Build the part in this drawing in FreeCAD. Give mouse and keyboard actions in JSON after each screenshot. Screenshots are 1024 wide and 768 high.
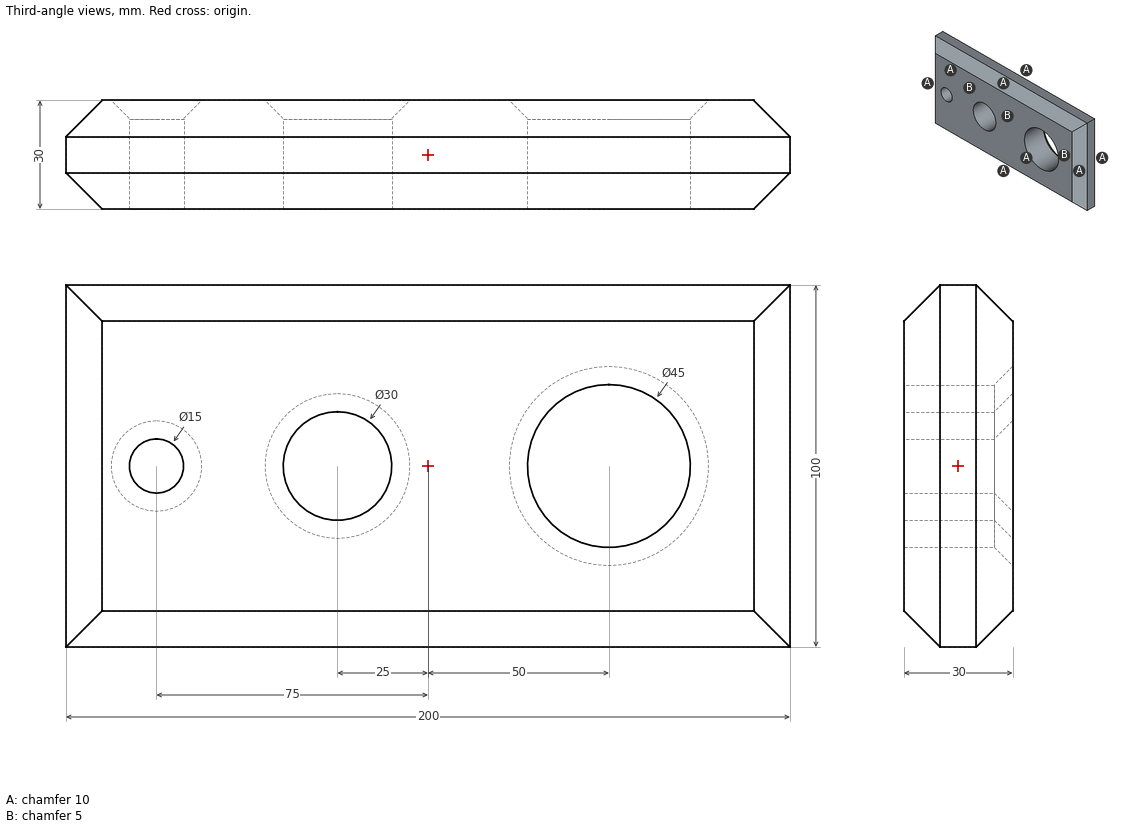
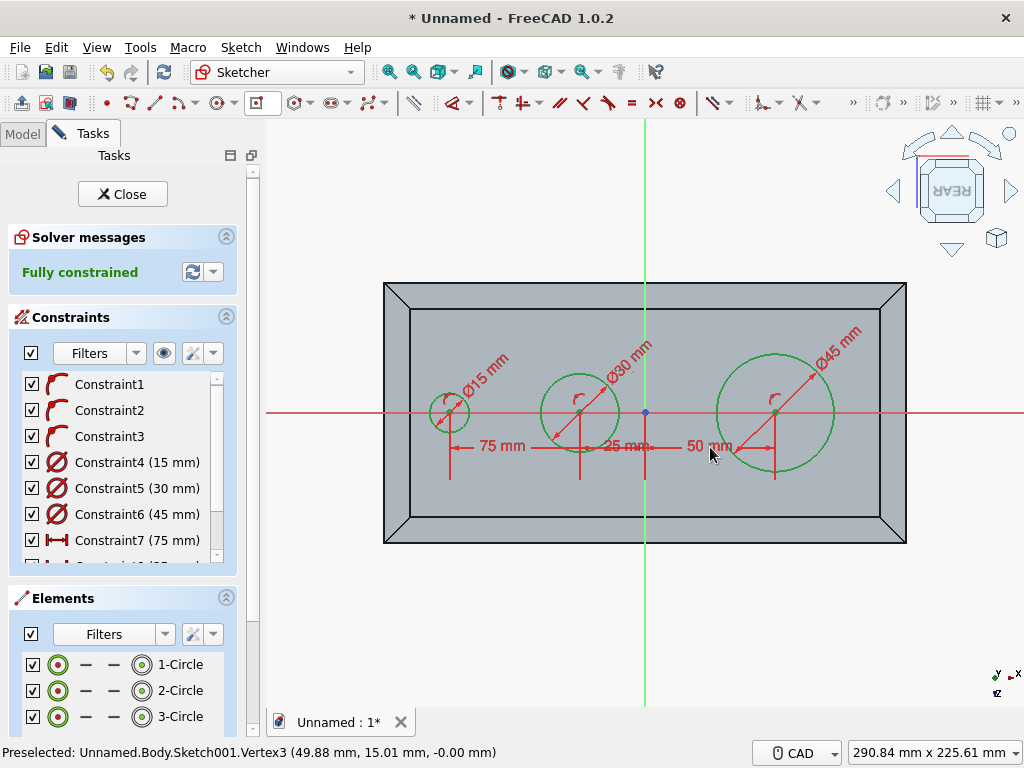
{"action": "left_click", "coordinate": [123, 194]}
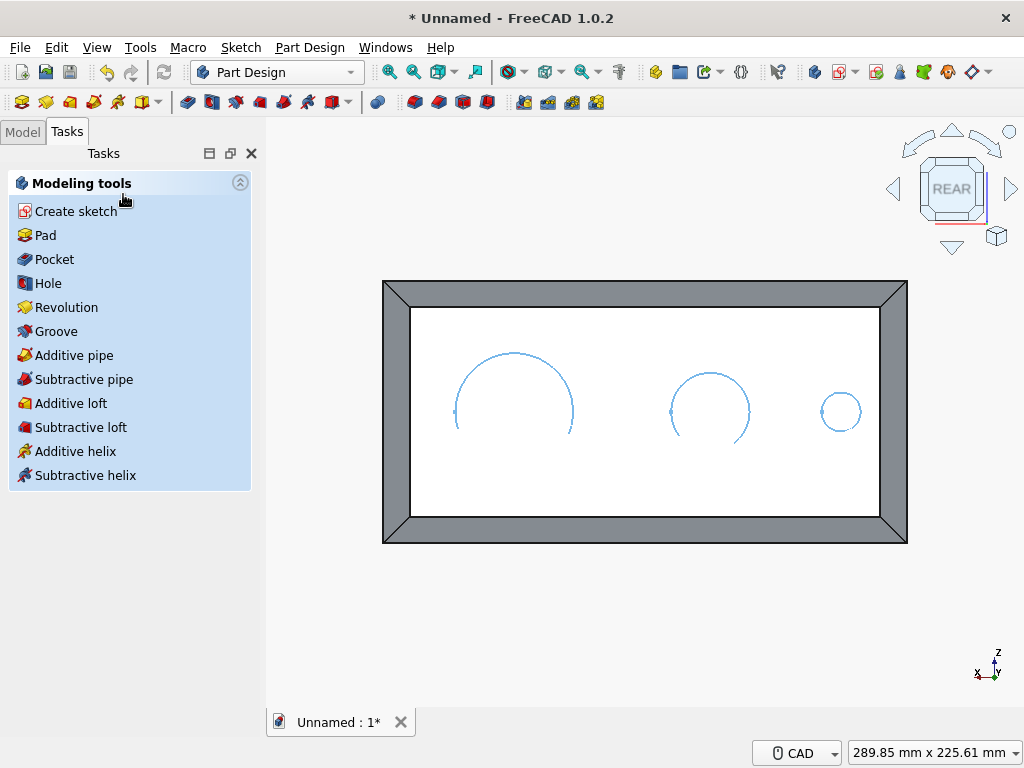
{"action": "left_click", "coordinate": [188, 102]}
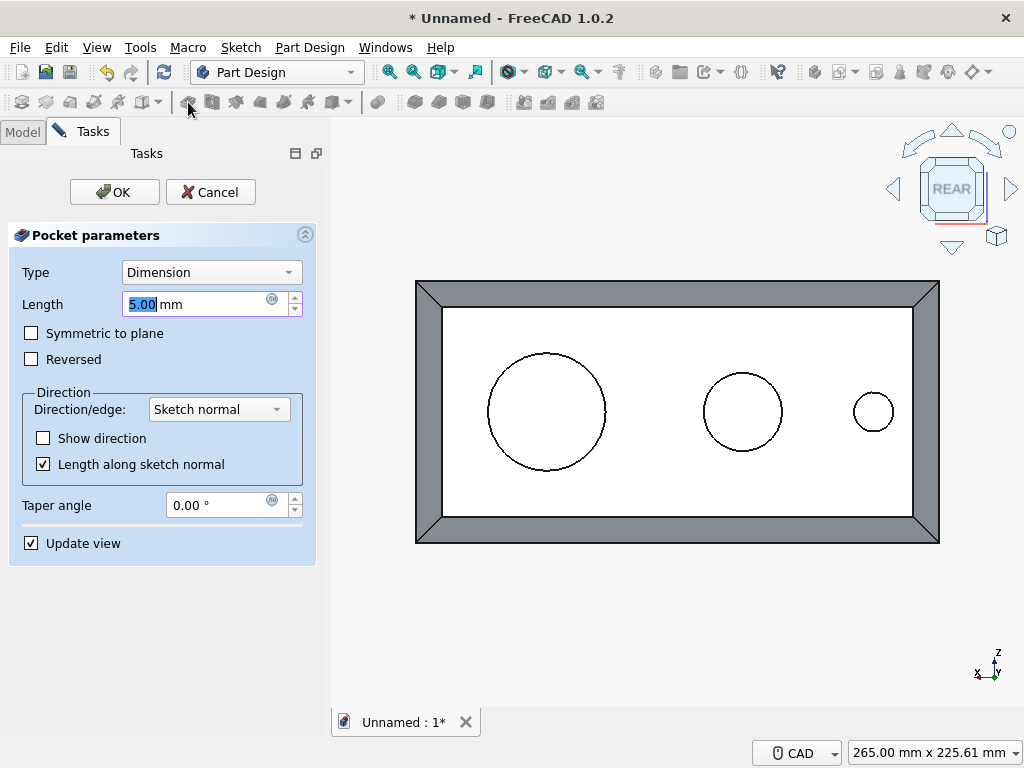
{"action": "type", "text": "30"}
{"action": "key", "text": "Tab"}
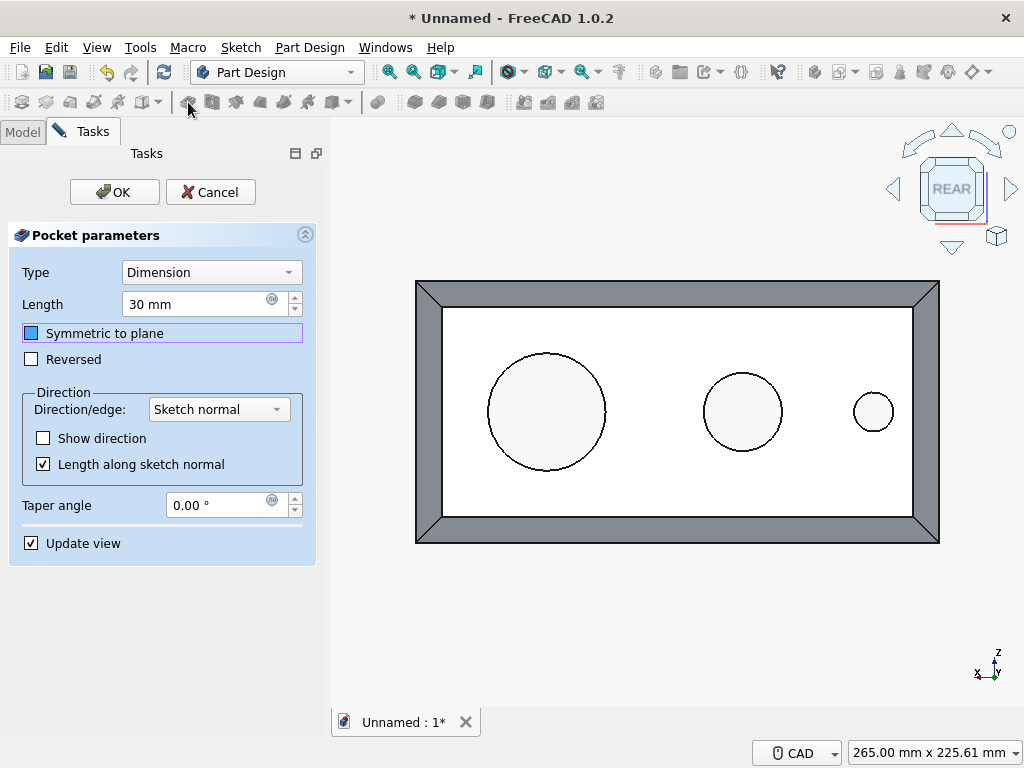
{"action": "left_click", "coordinate": [115, 192]}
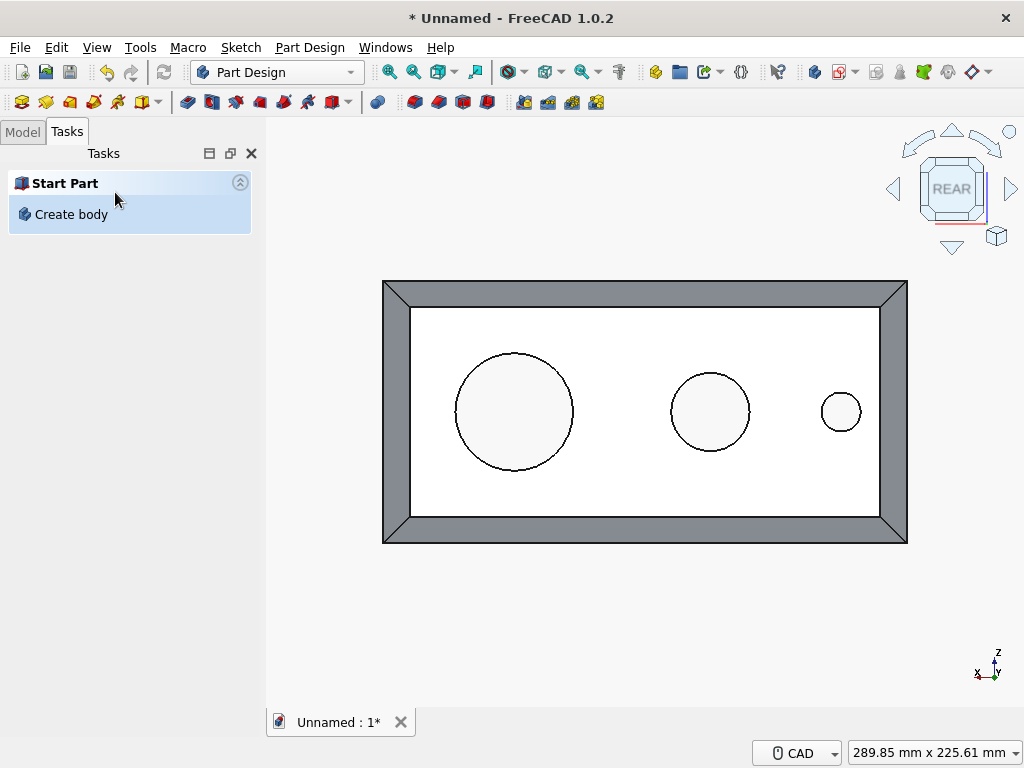
{"action": "left_click", "coordinate": [861, 411]}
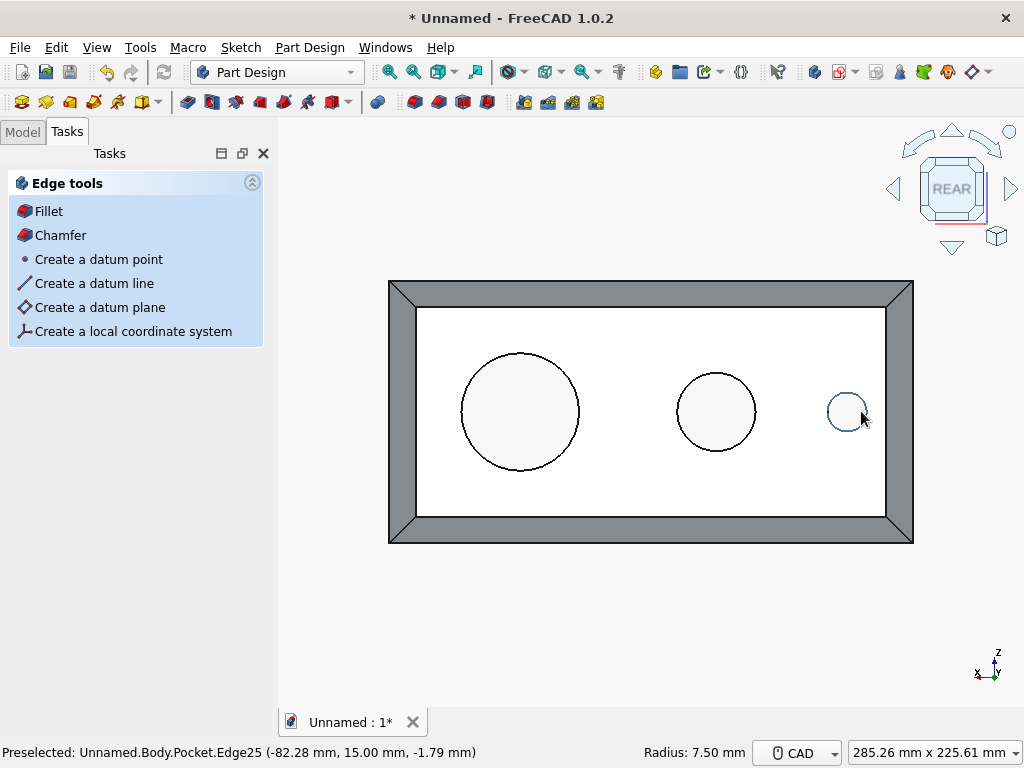
{"action": "left_click", "coordinate": [748, 388], "text": "ctrl"}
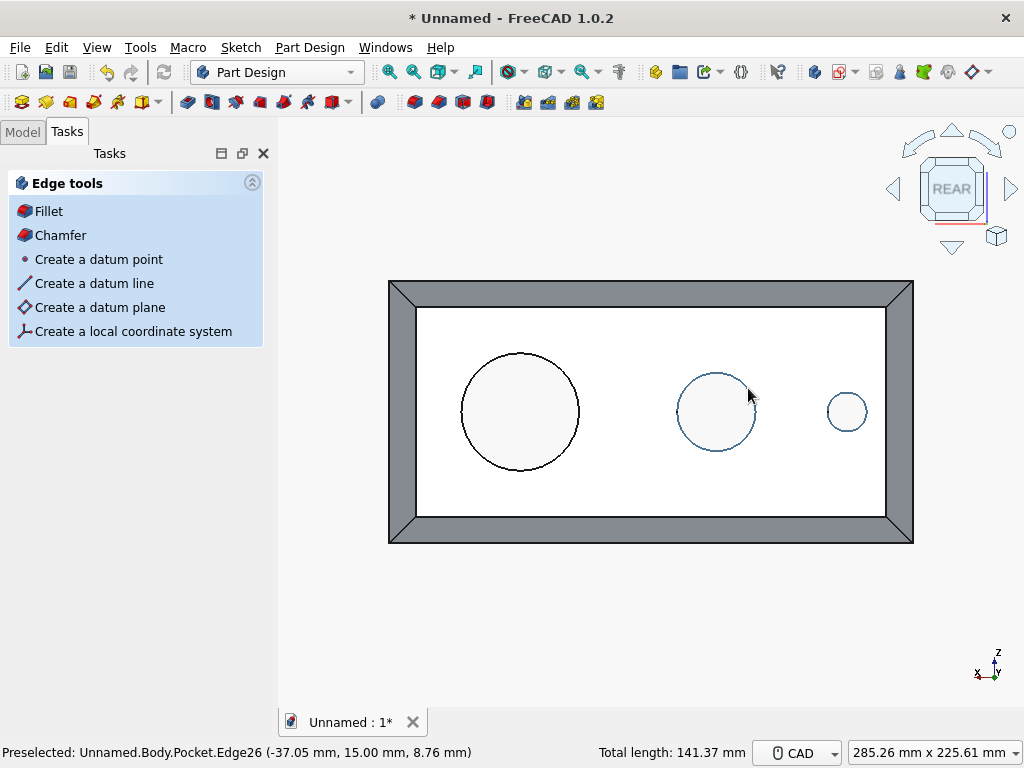
{"action": "left_click", "coordinate": [568, 376], "text": "ctrl"}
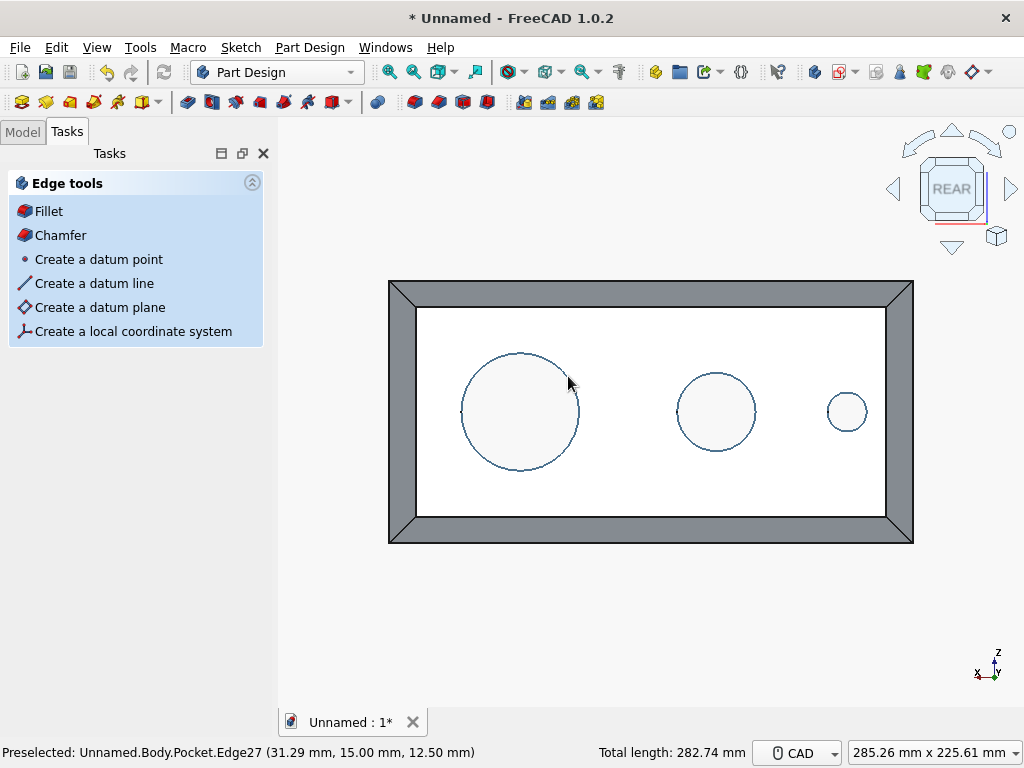
{"action": "left_click", "coordinate": [440, 102]}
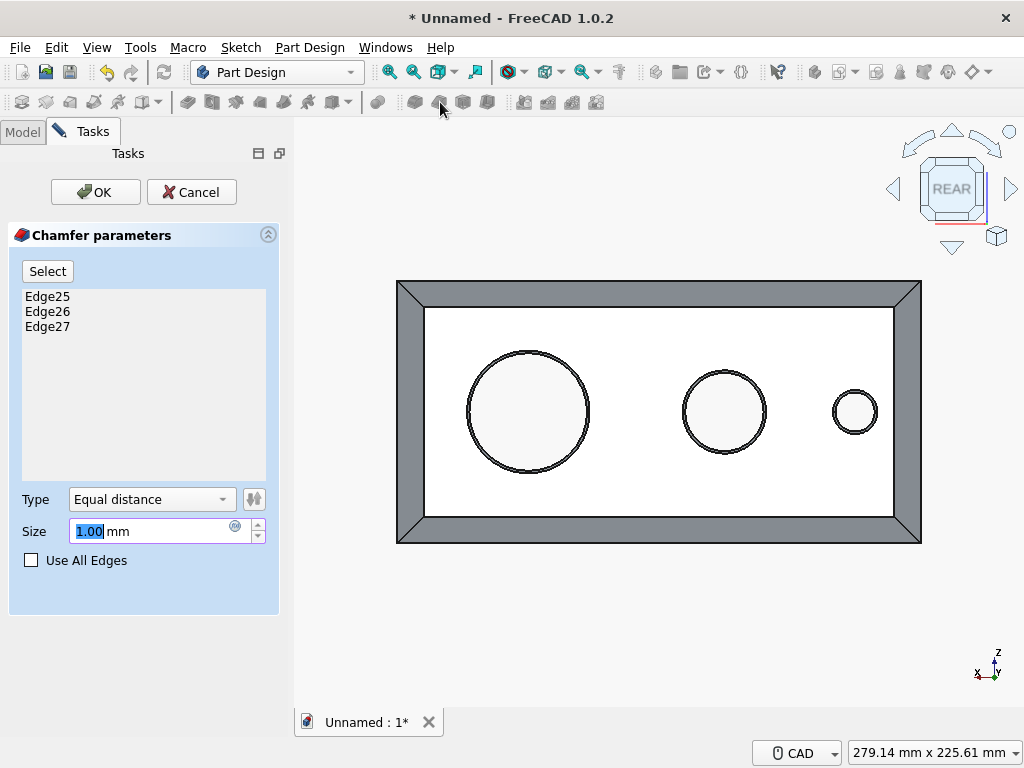
{"action": "type", "text": "5"}
{"action": "key", "text": "Tab"}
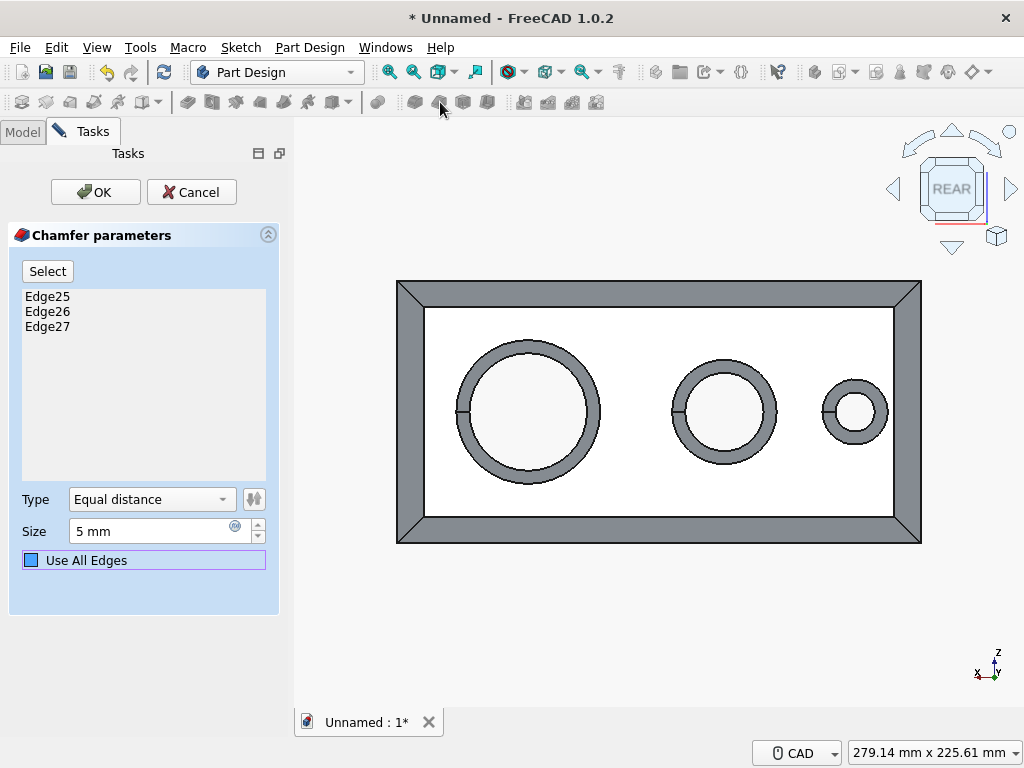
{"action": "left_click", "coordinate": [96, 192]}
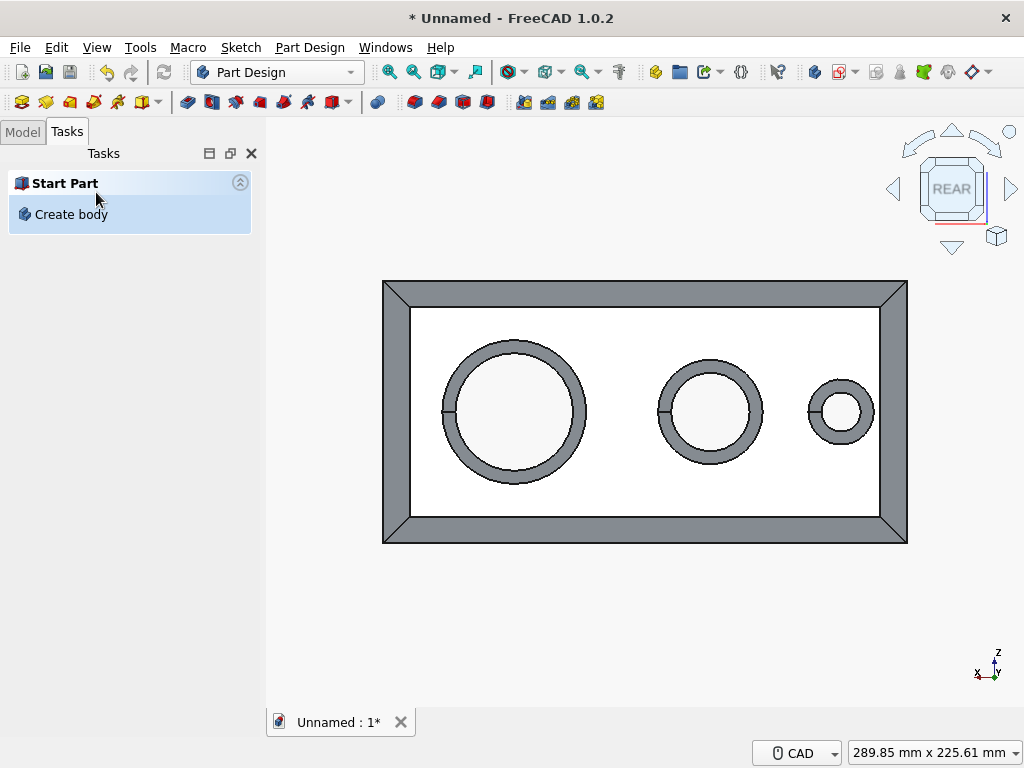
{"action": "key", "text": "0"}